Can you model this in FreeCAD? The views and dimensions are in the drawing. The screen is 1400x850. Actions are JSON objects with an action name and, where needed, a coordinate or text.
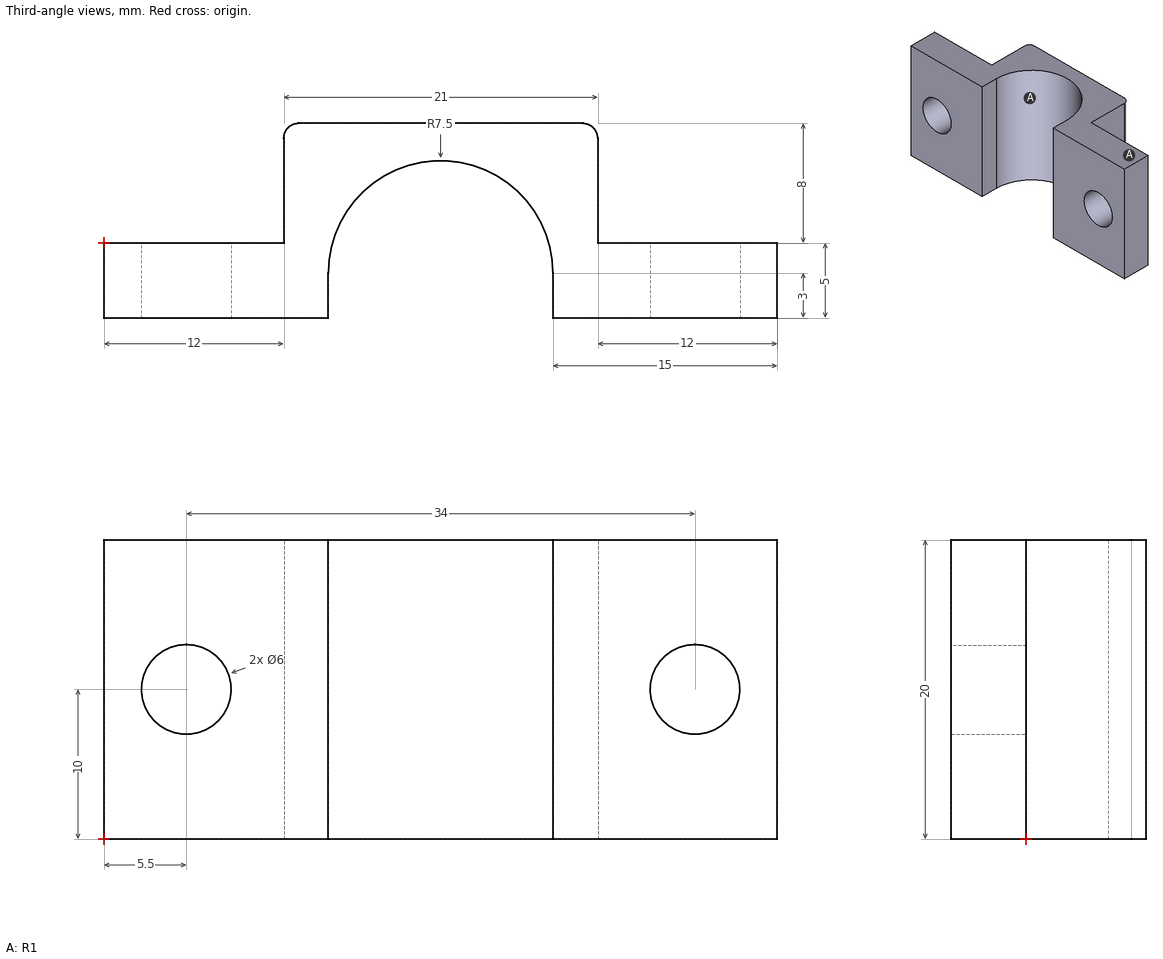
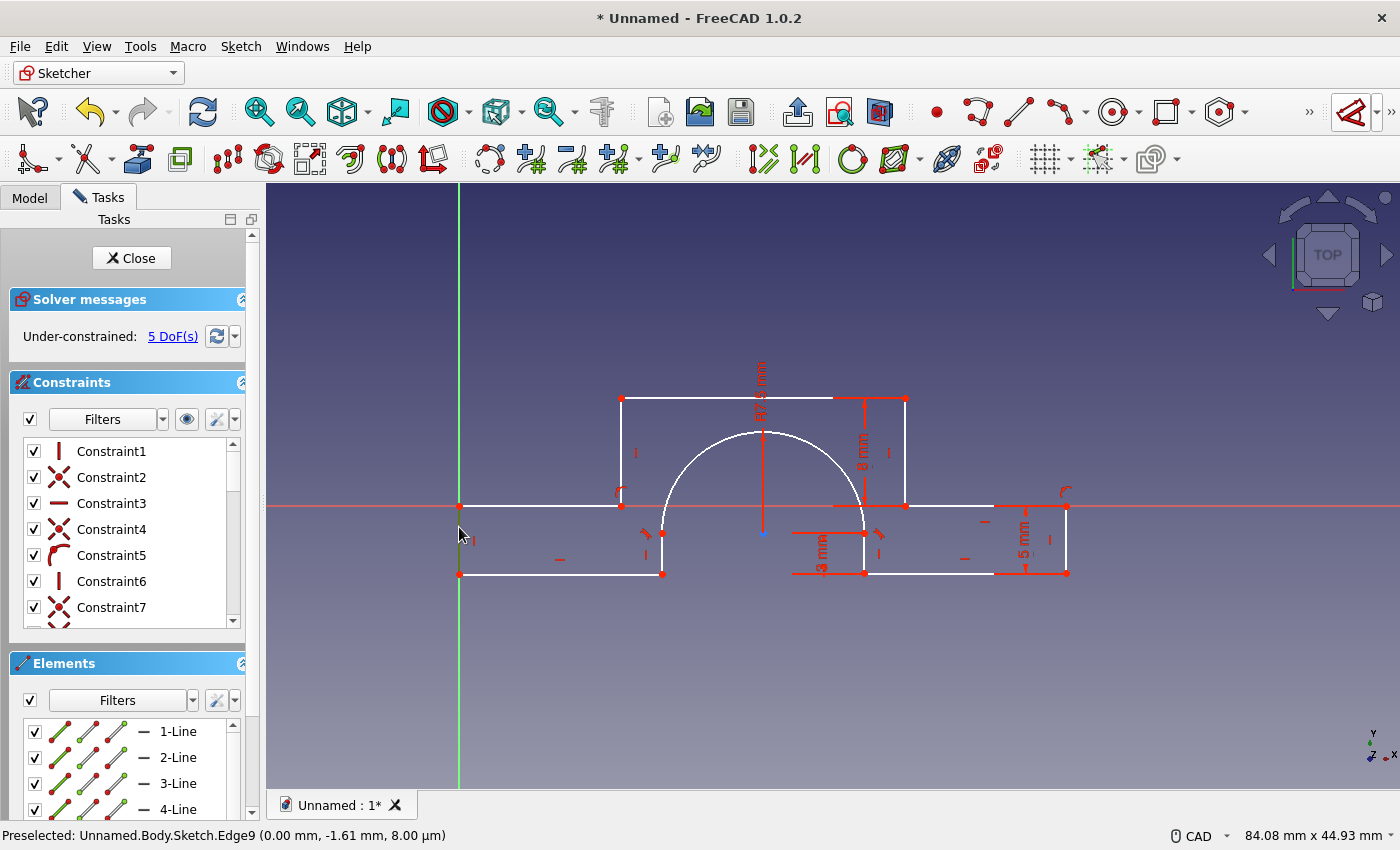
{"action": "left_click", "coordinate": [1376, 112]}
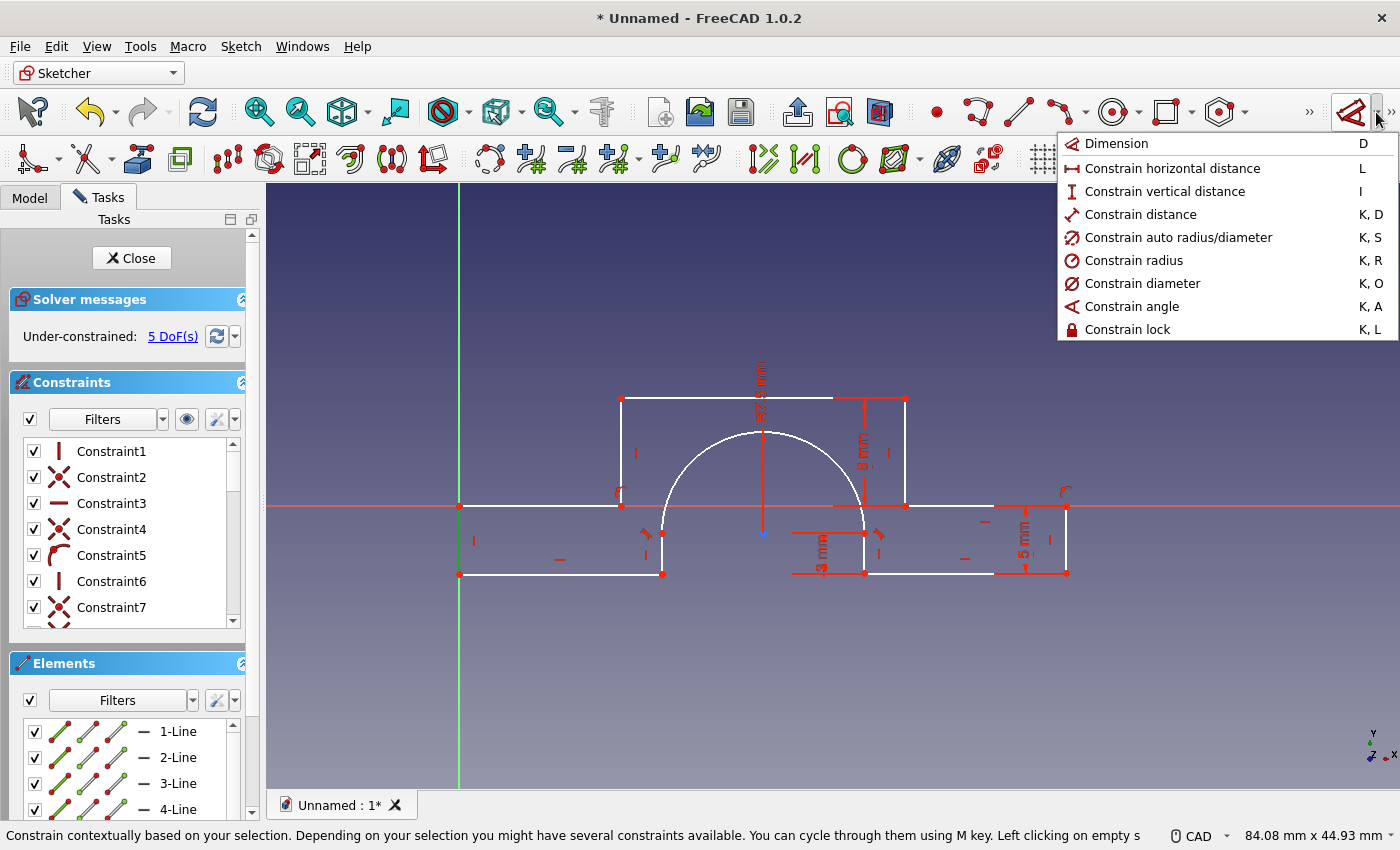
{"action": "left_click", "coordinate": [1228, 192]}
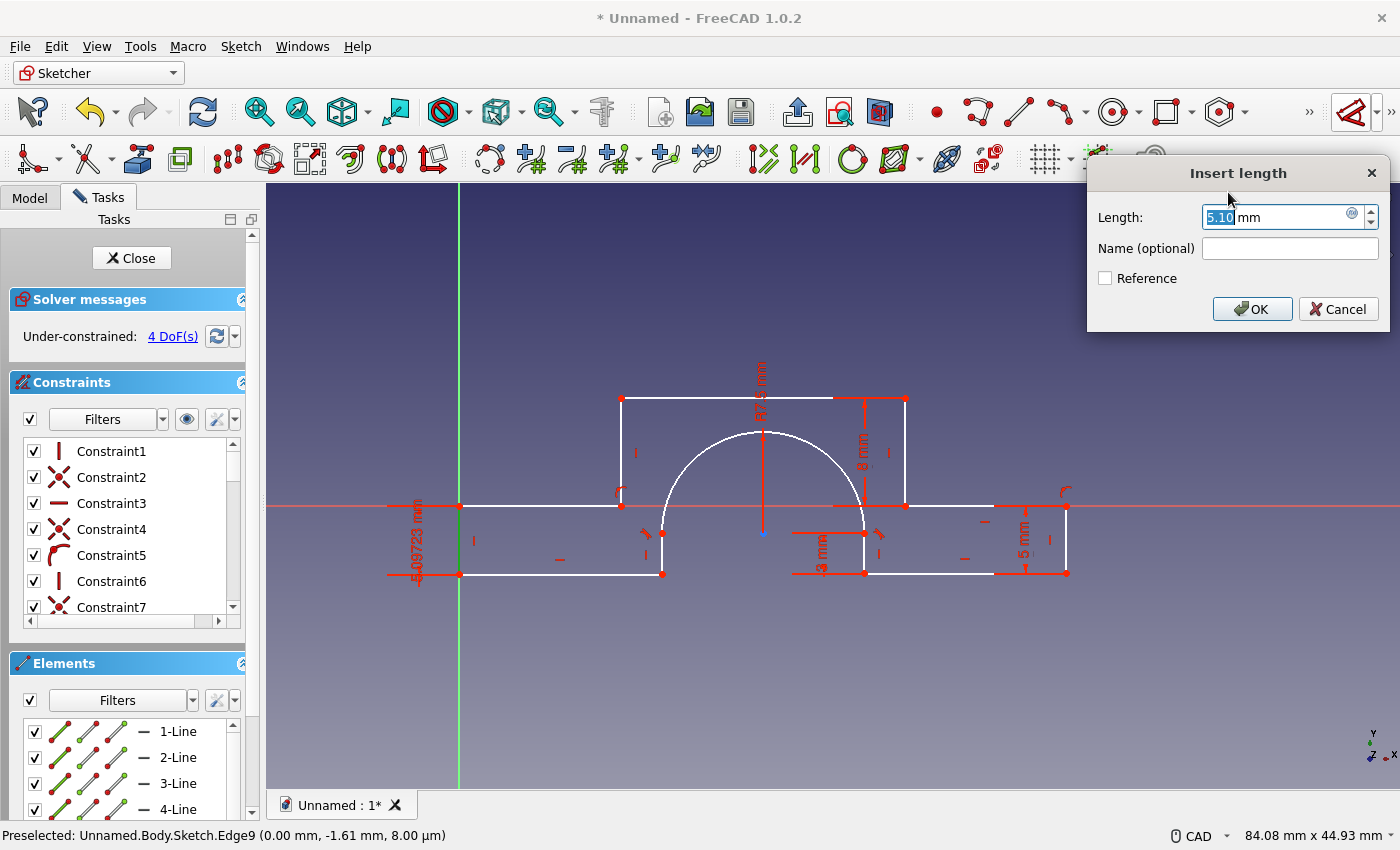
{"action": "type", "text": "5"}
{"action": "key", "text": "Return"}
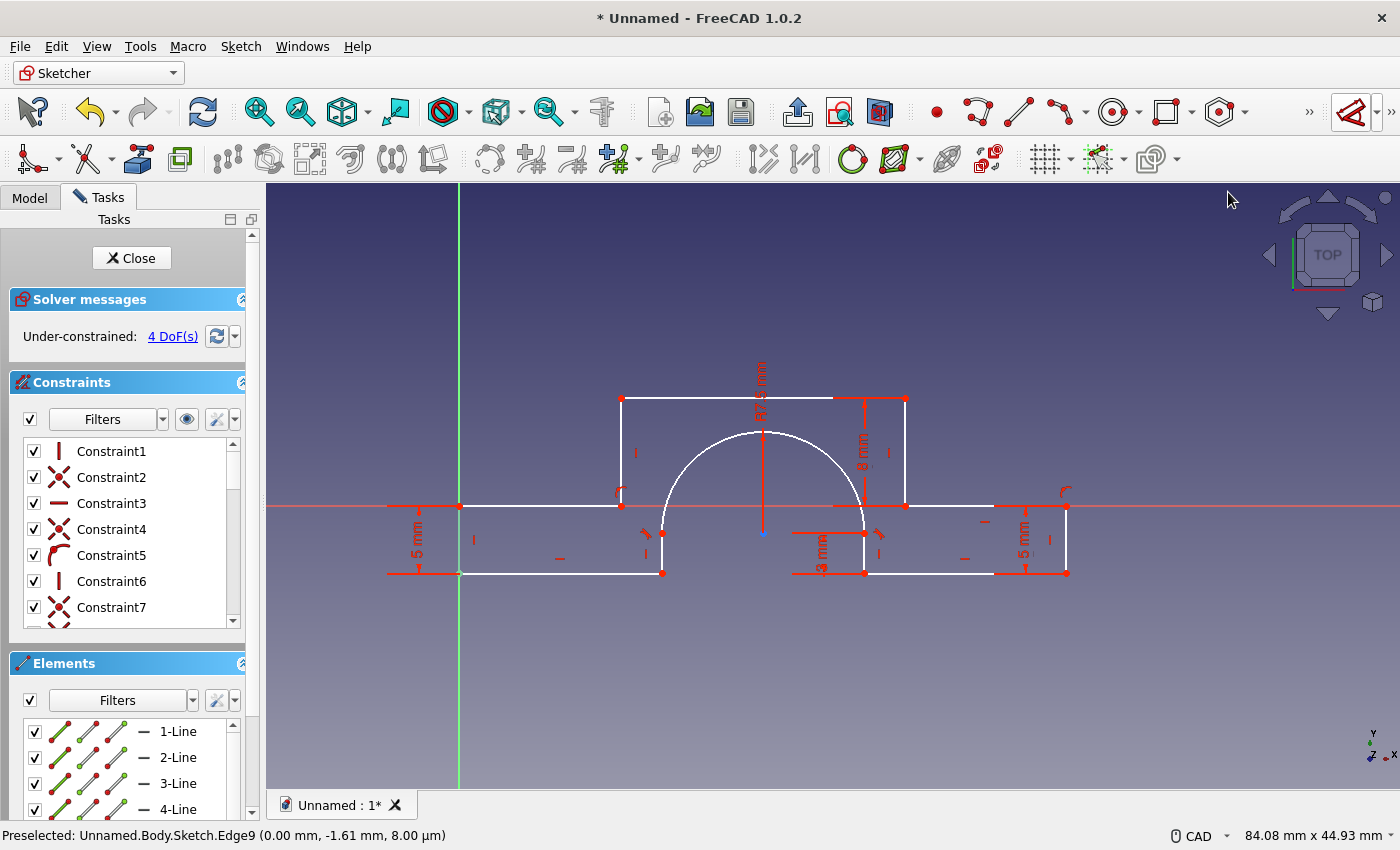
{"action": "left_click", "coordinate": [925, 574]}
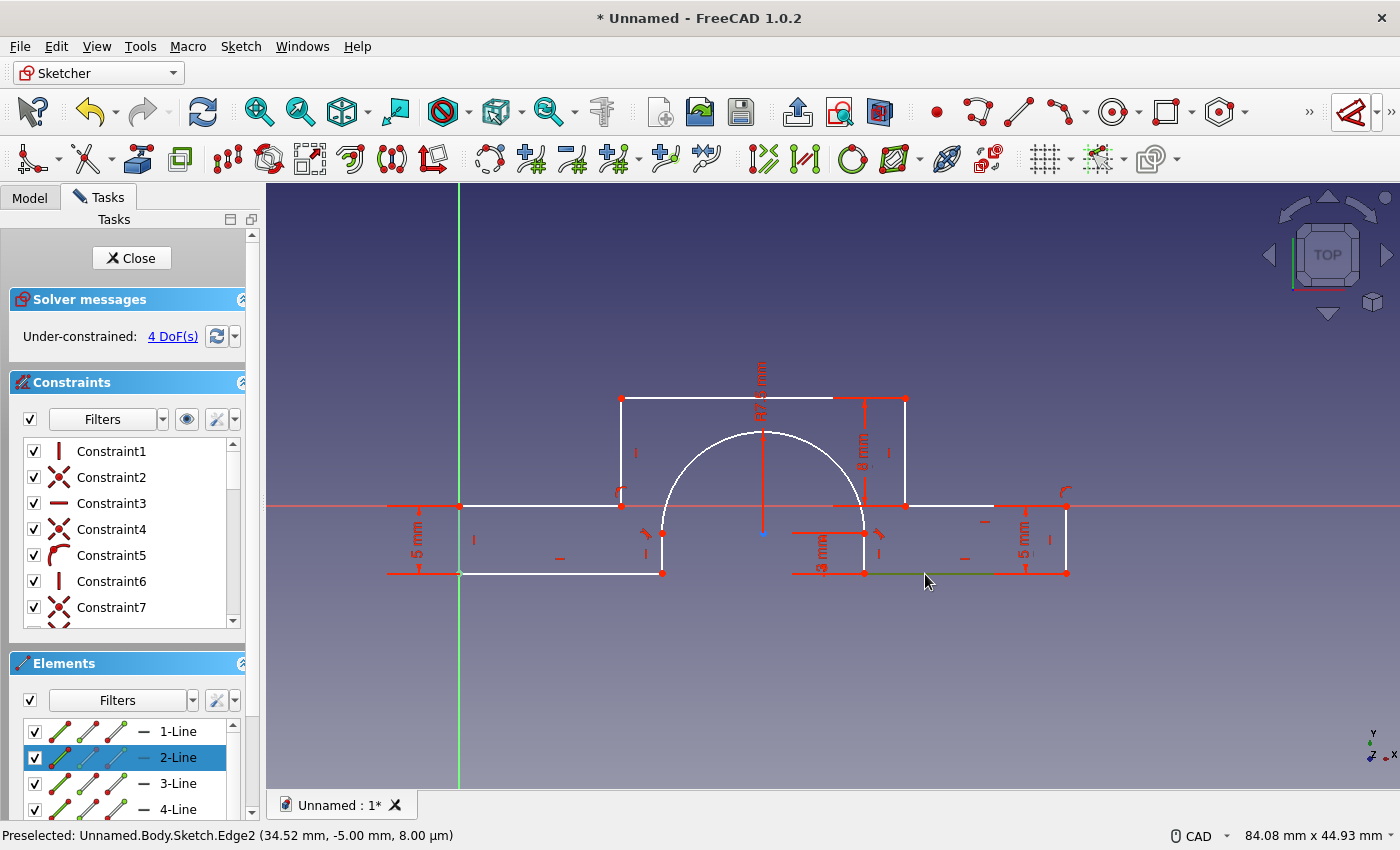
{"action": "key", "text": "l"}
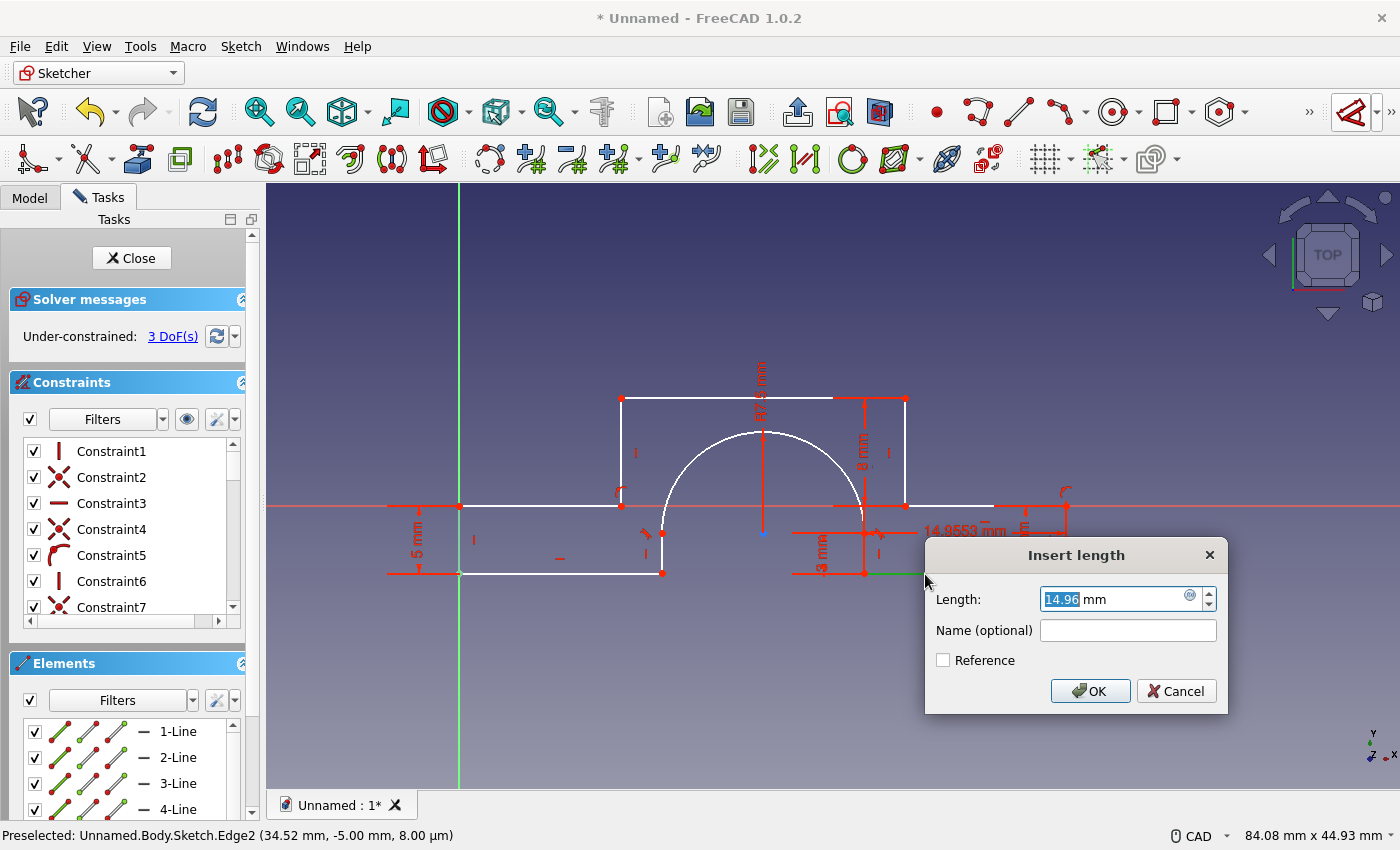
{"action": "type", "text": "15"}
{"action": "key", "text": "Return"}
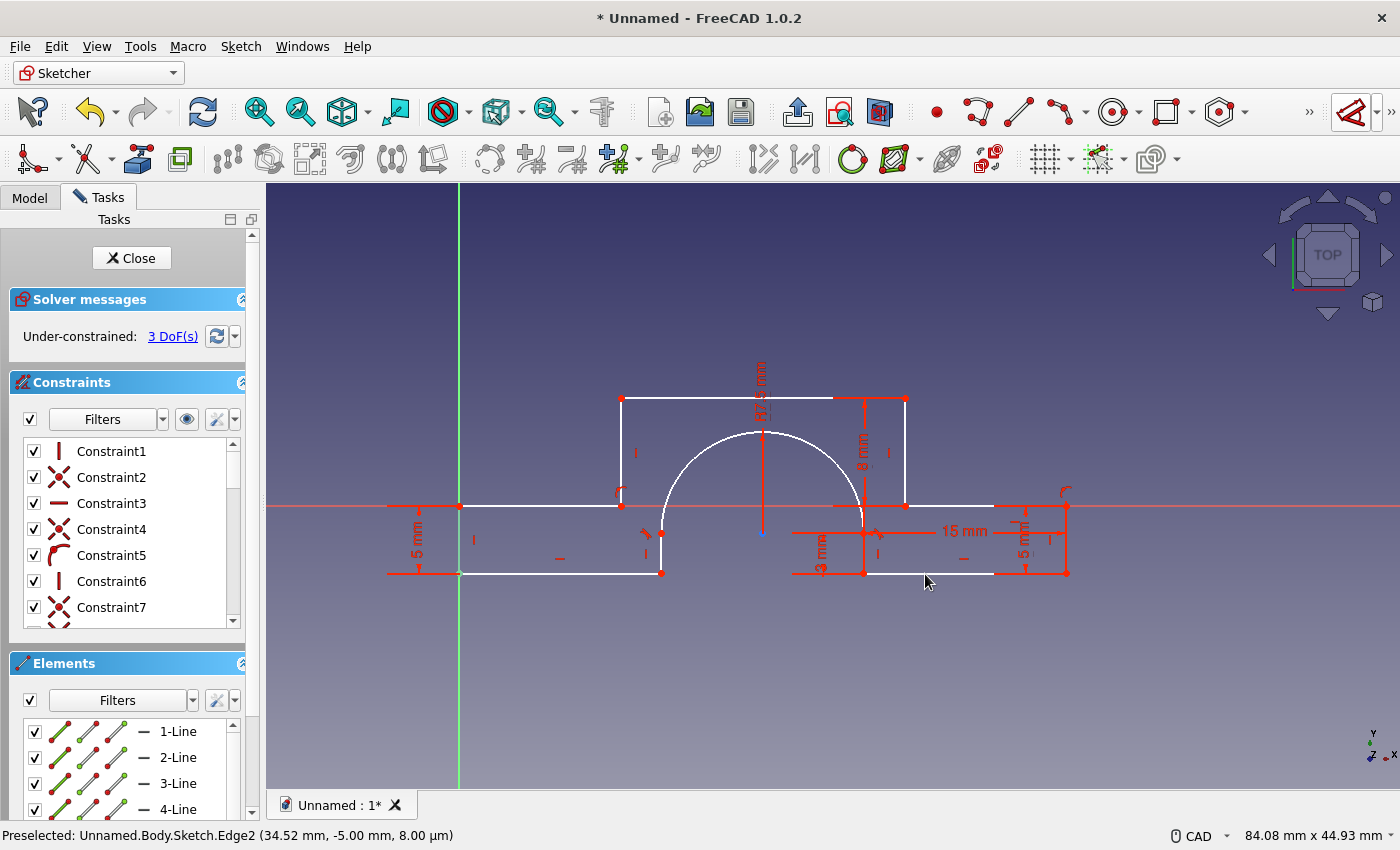
{"action": "left_click", "coordinate": [1018, 506]}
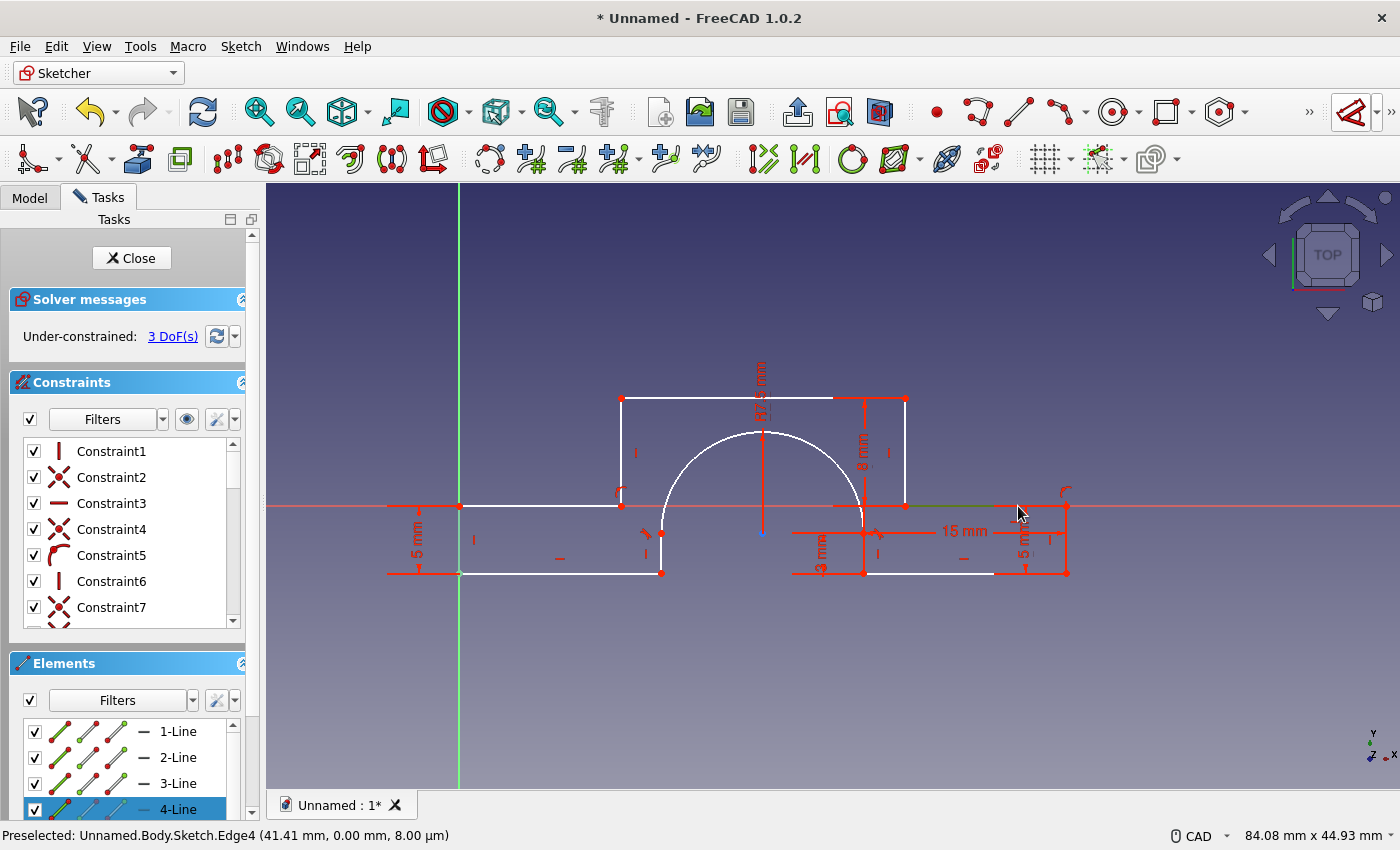
{"action": "left_click", "coordinate": [1376, 112]}